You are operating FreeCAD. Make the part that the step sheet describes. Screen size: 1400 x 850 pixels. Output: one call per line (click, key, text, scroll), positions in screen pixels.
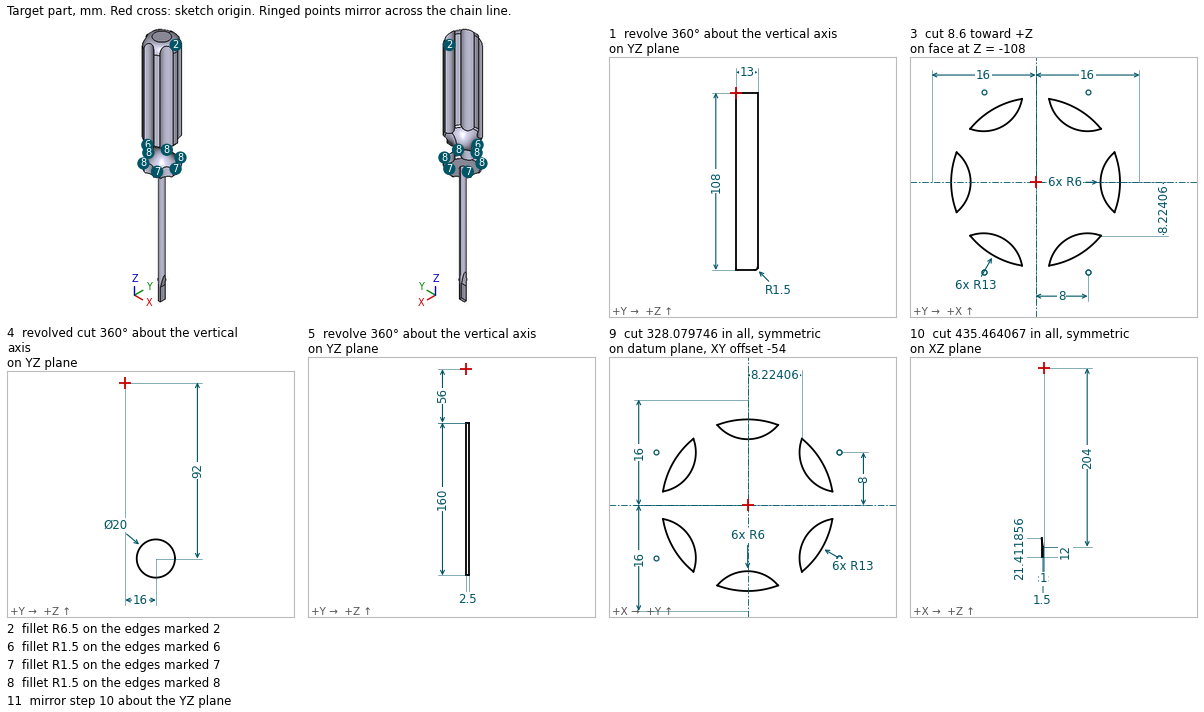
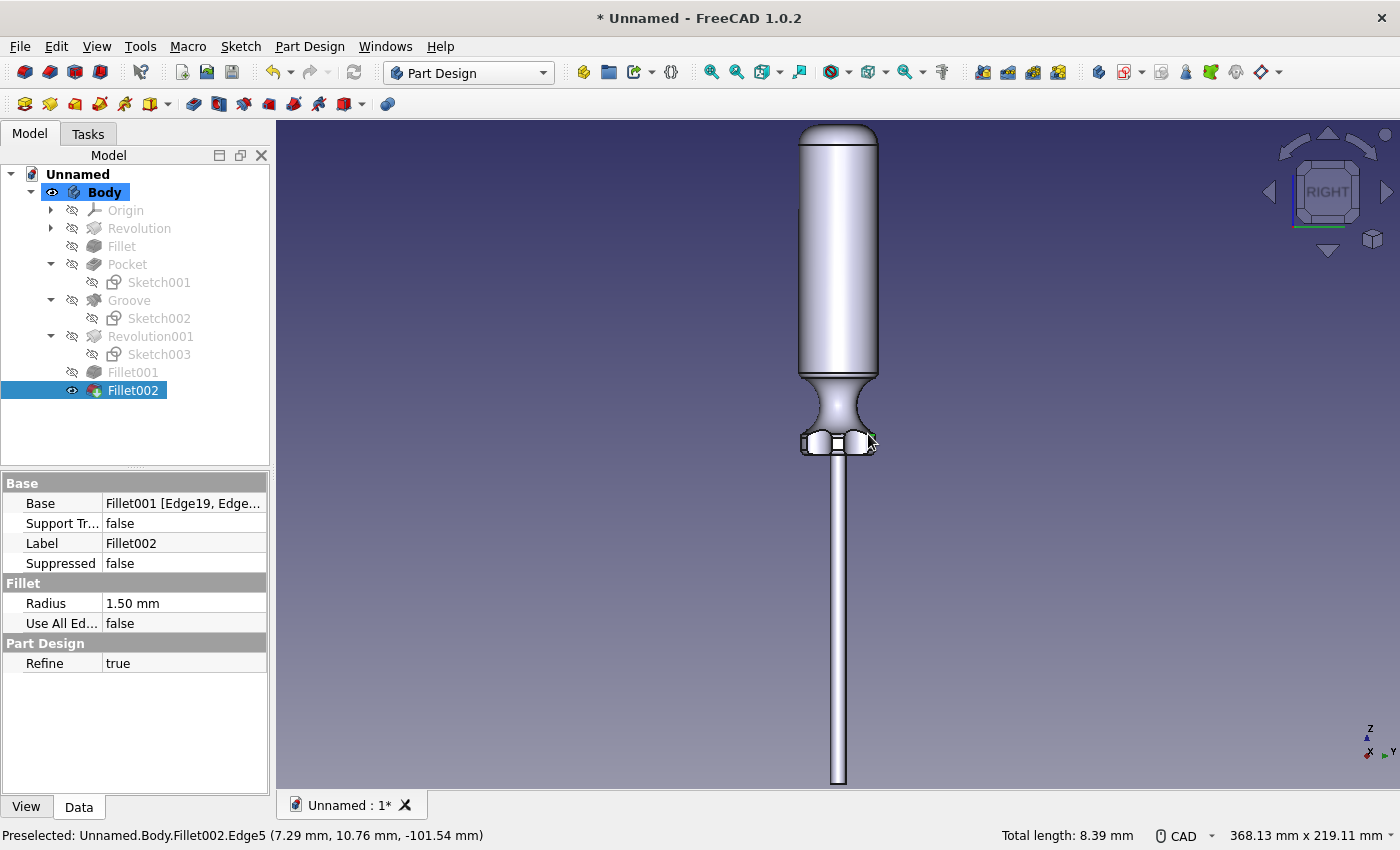
key(5)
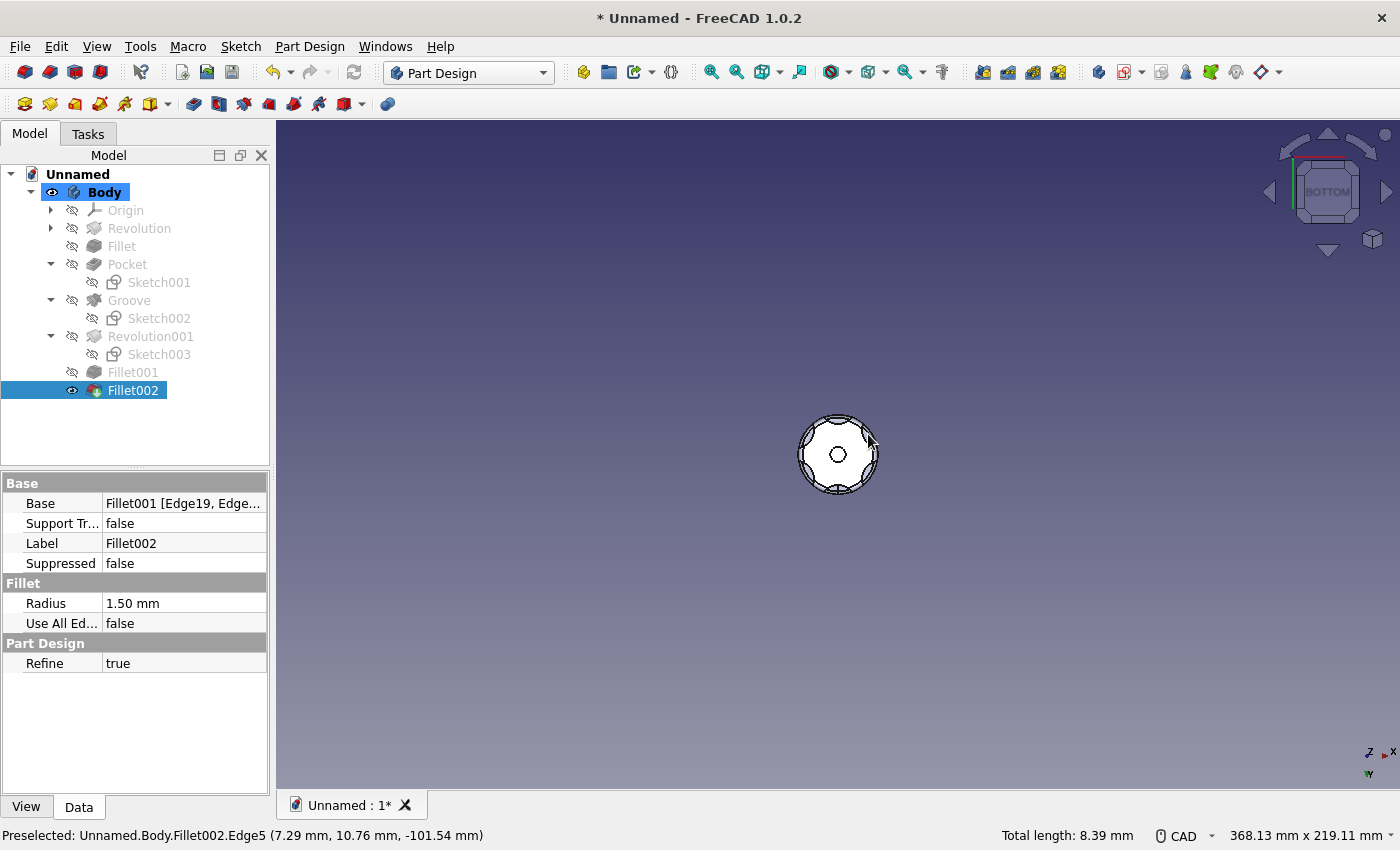
key(v)
key(f)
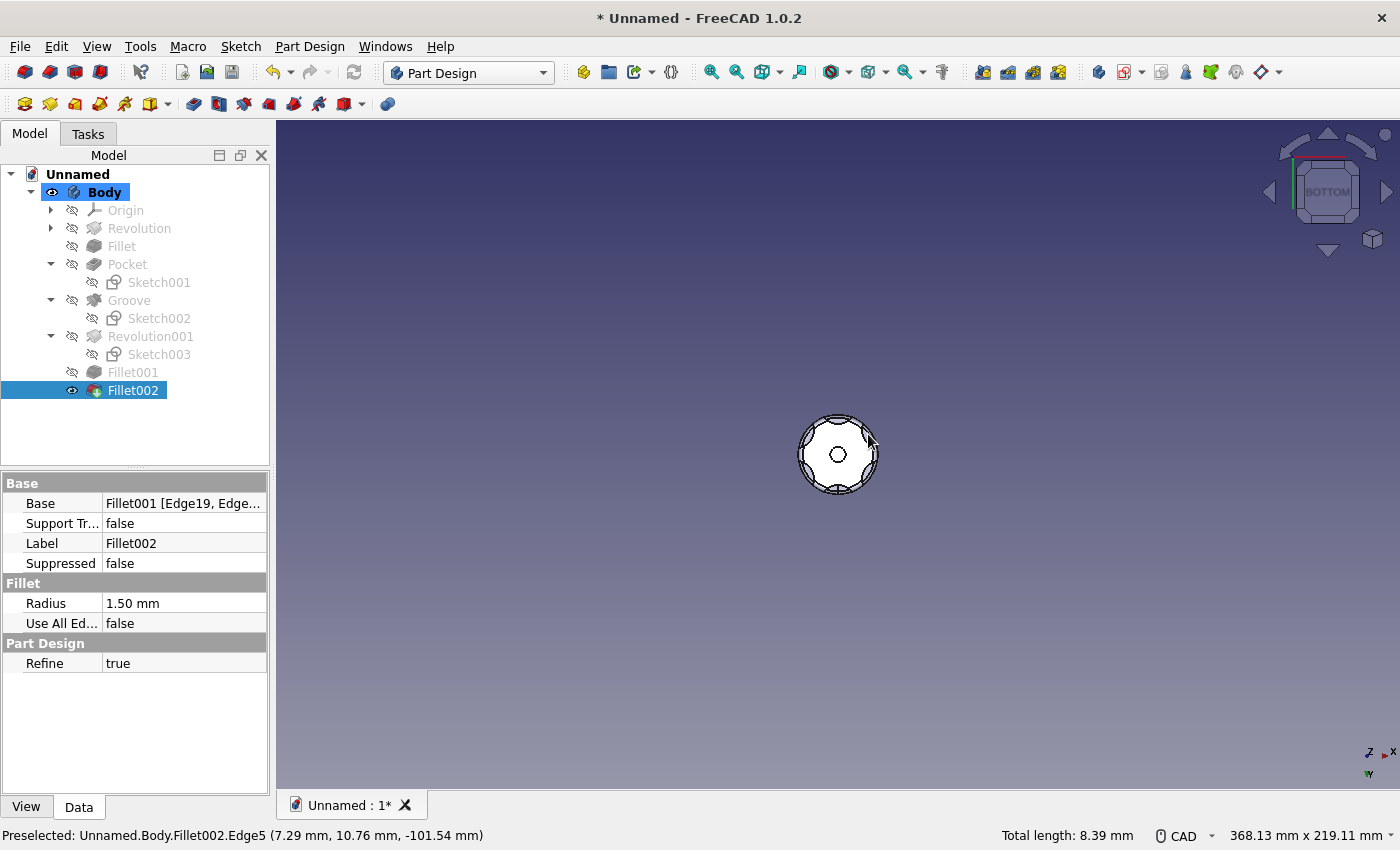
scroll(818, 488, up, 6)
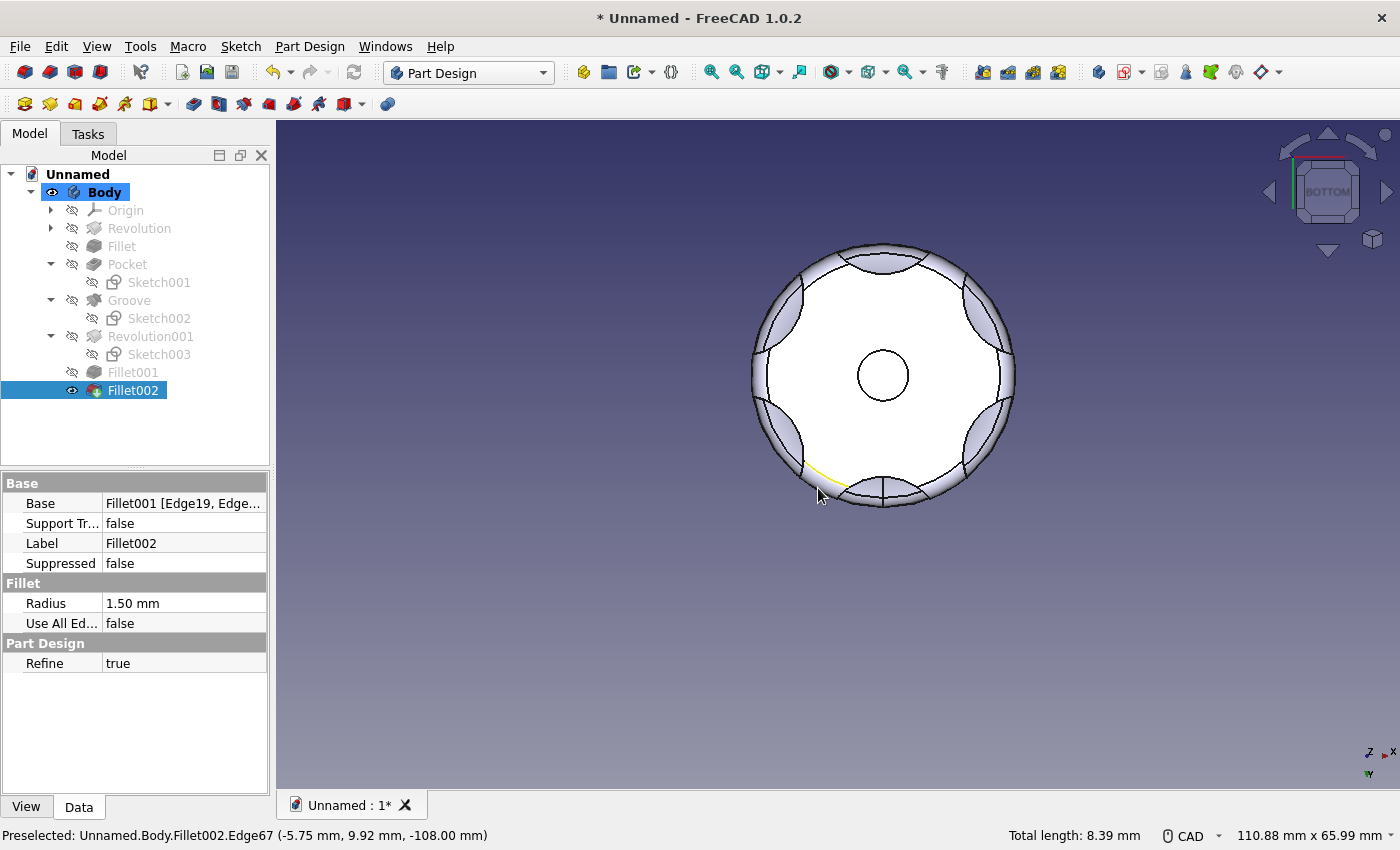
click(712, 72)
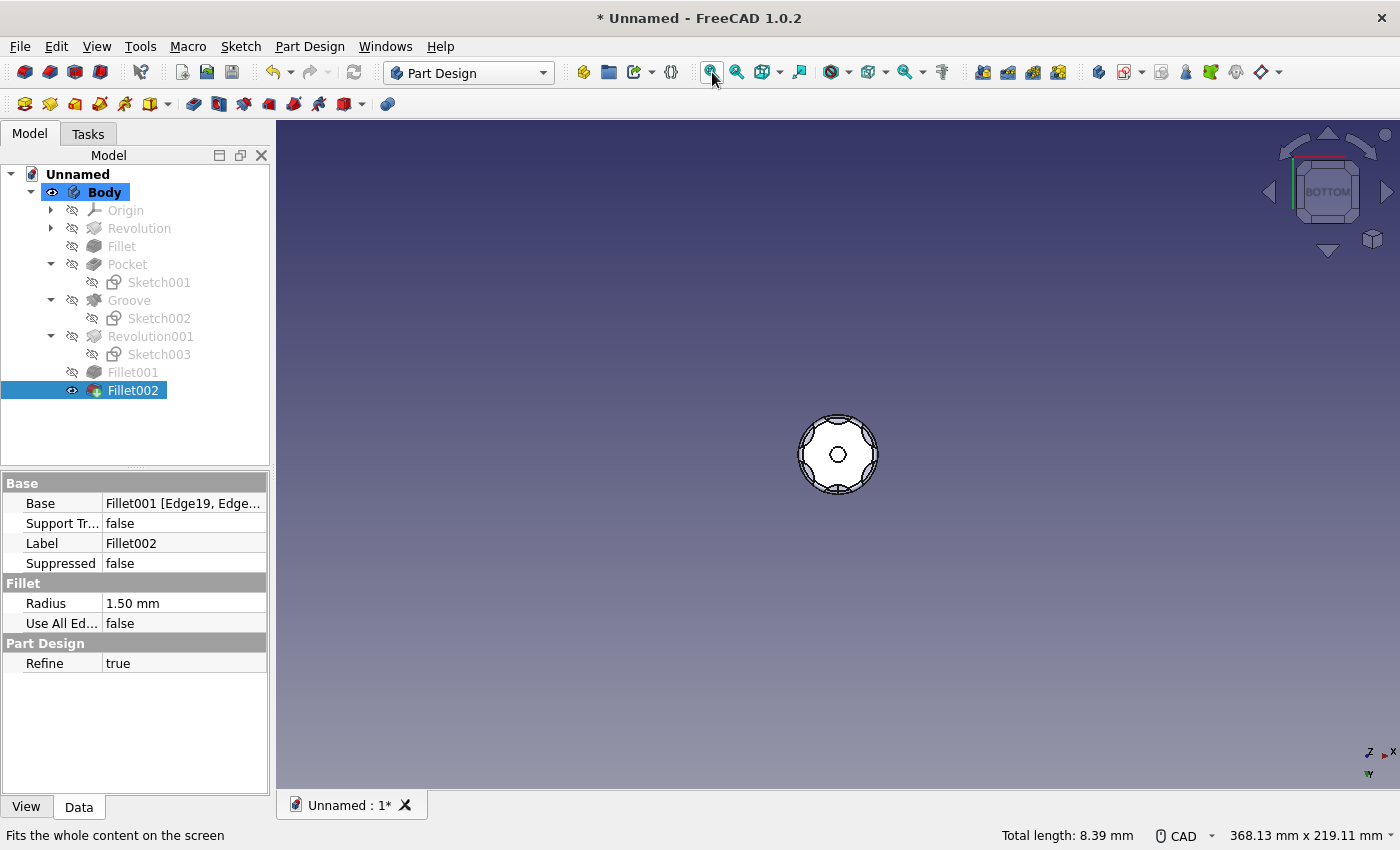
key(4)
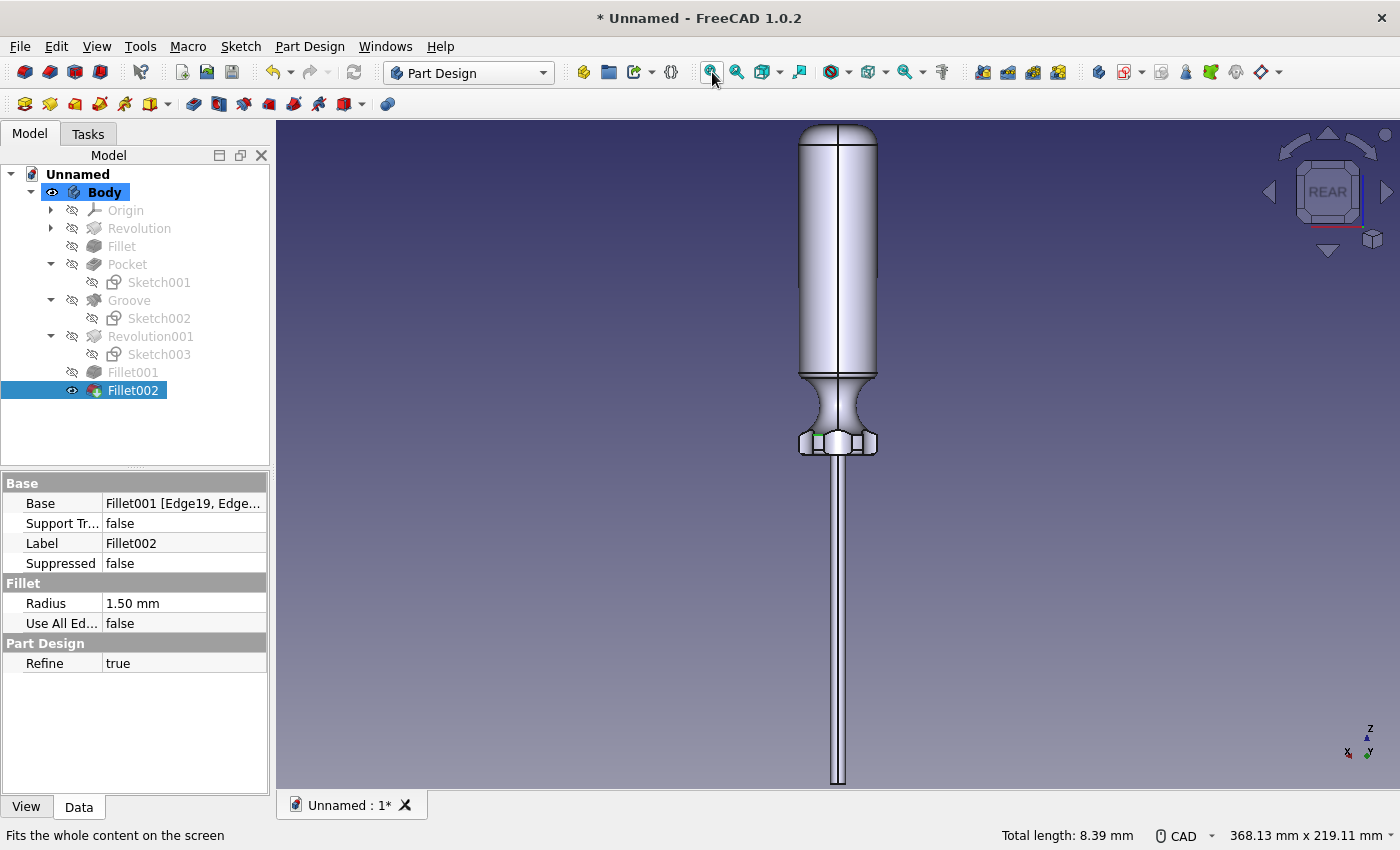
click(859, 434, ctrl)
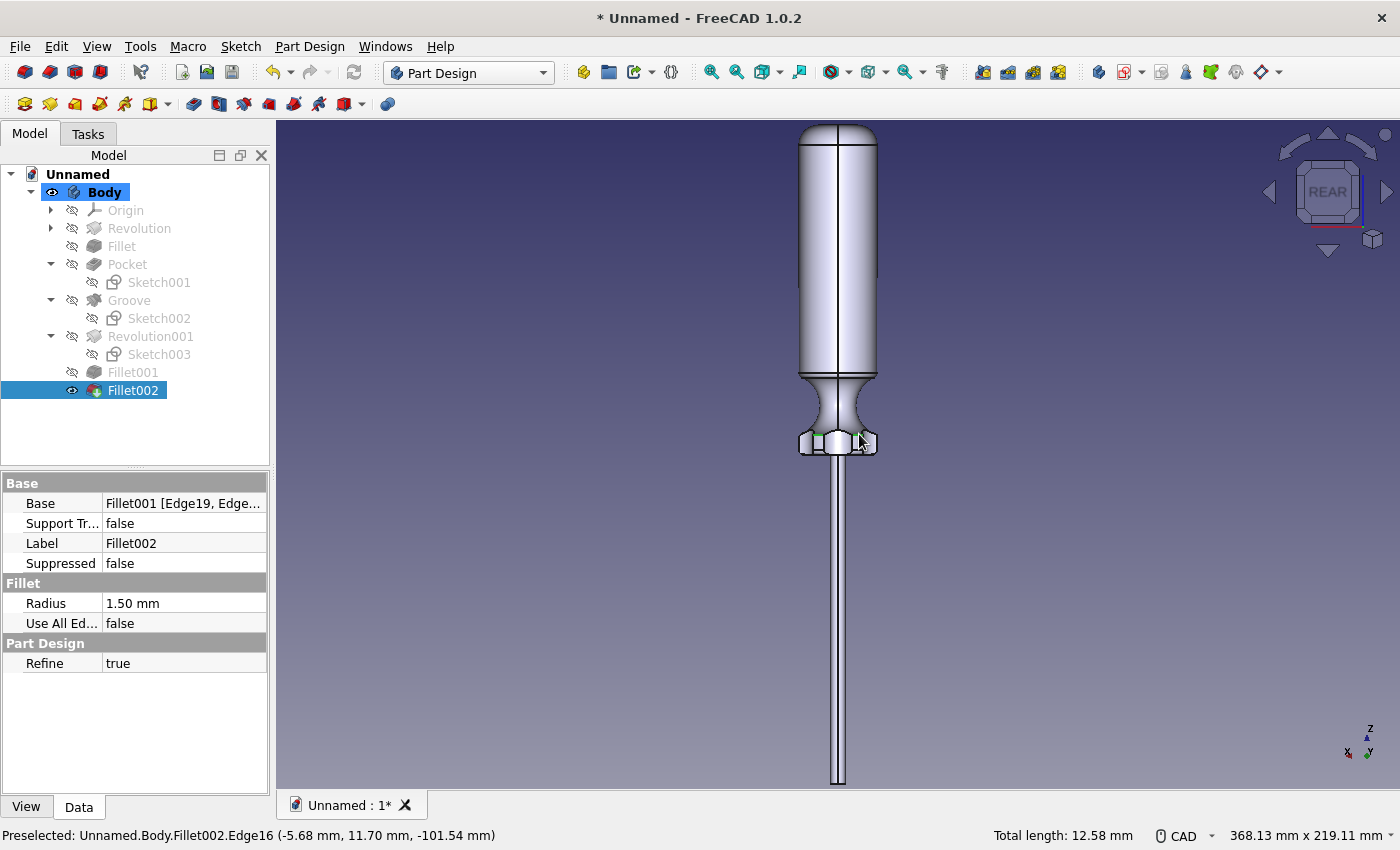
scroll(878, 434, up, 6)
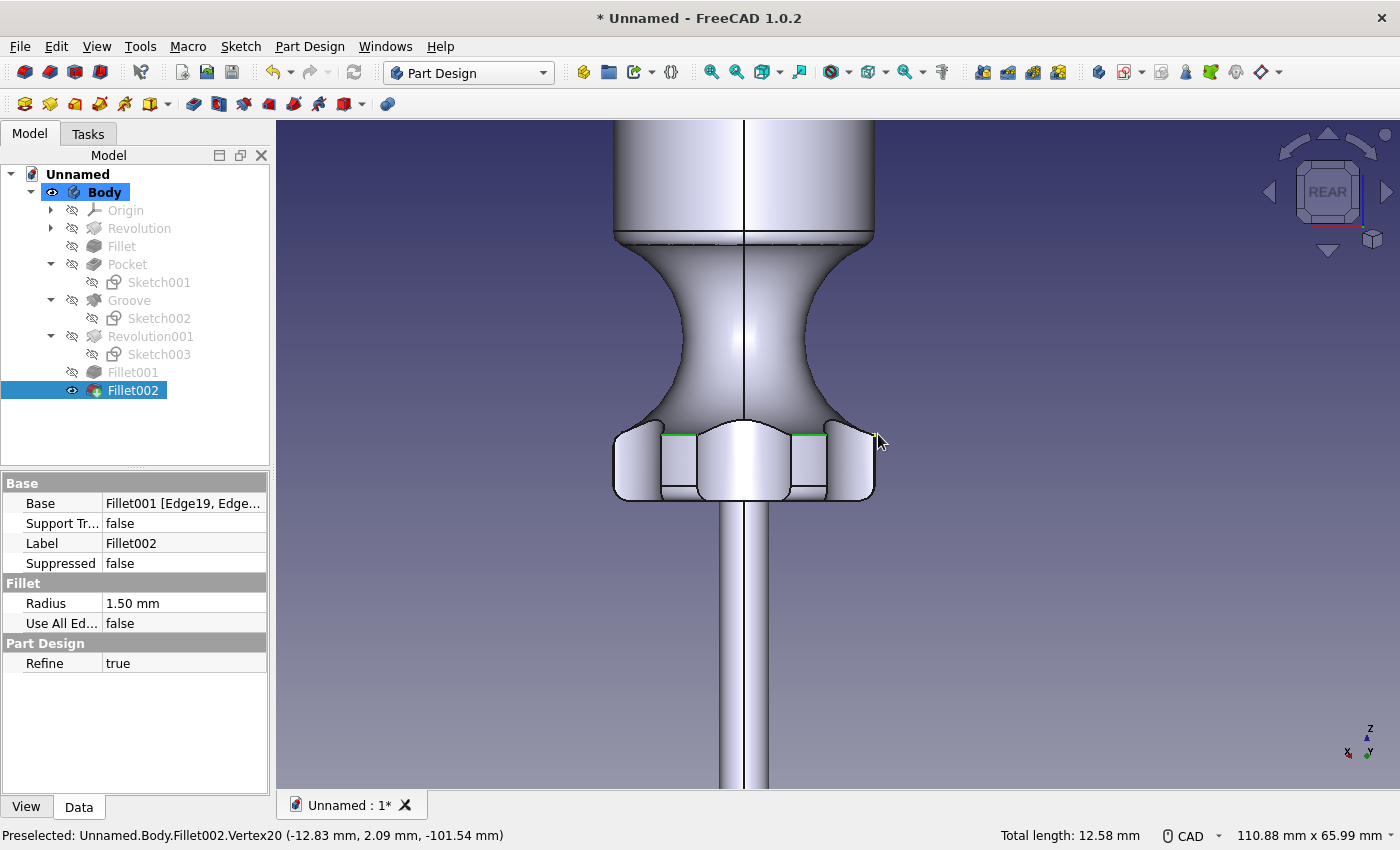
key(v)
key(f)